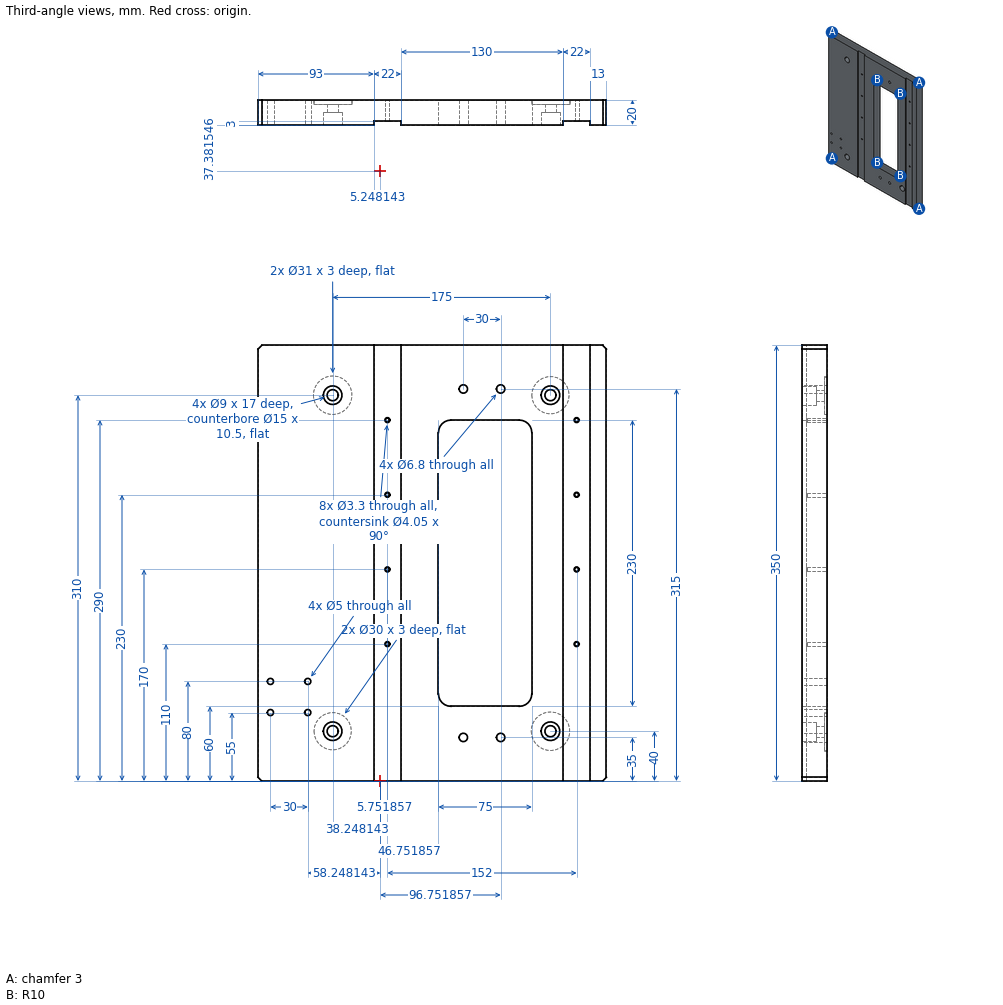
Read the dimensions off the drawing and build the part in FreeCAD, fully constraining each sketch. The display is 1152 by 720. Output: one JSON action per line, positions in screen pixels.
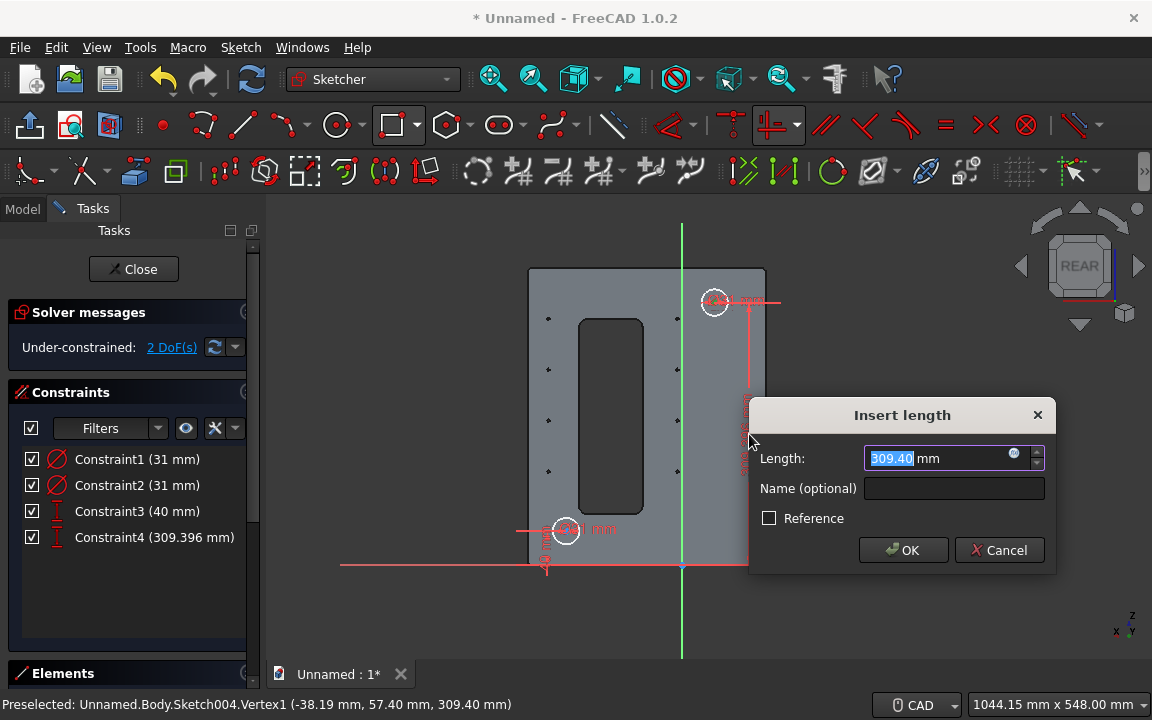
{"action": "type", "text": "310"}
{"action": "key", "text": "Return"}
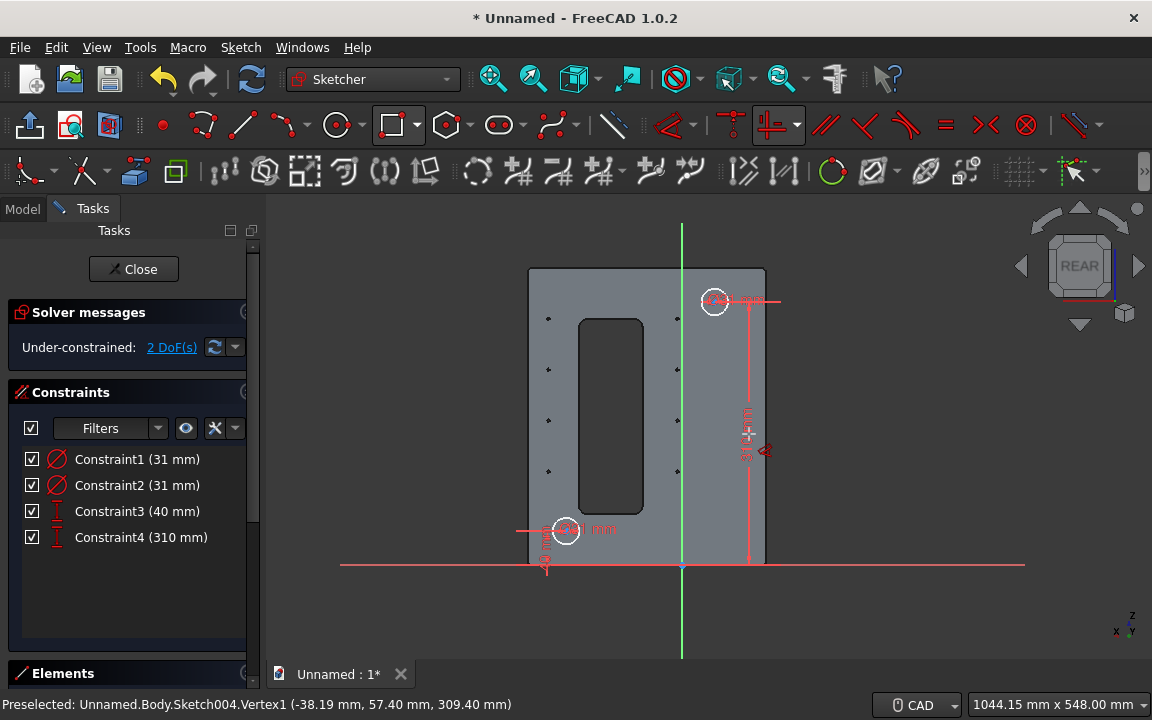
{"action": "left_click", "coordinate": [715, 302]}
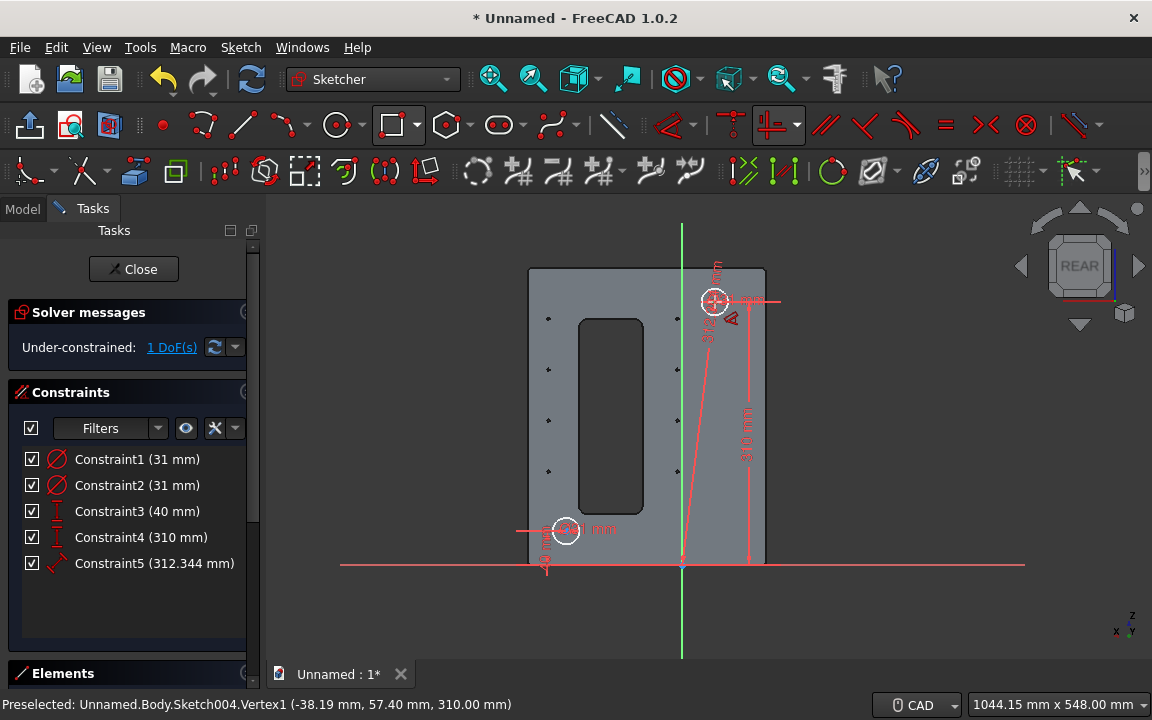
{"action": "left_click", "coordinate": [566, 531]}
{"action": "left_click", "coordinate": [640, 268]}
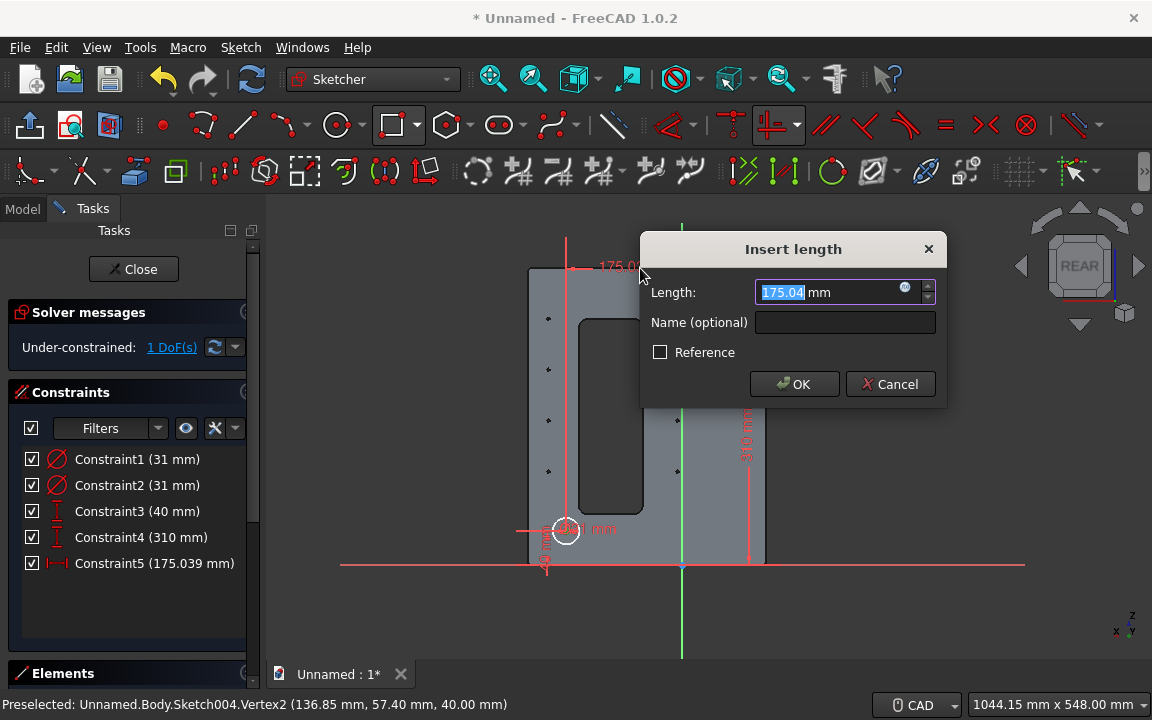
{"action": "type", "text": "175"}
{"action": "key", "text": "Return"}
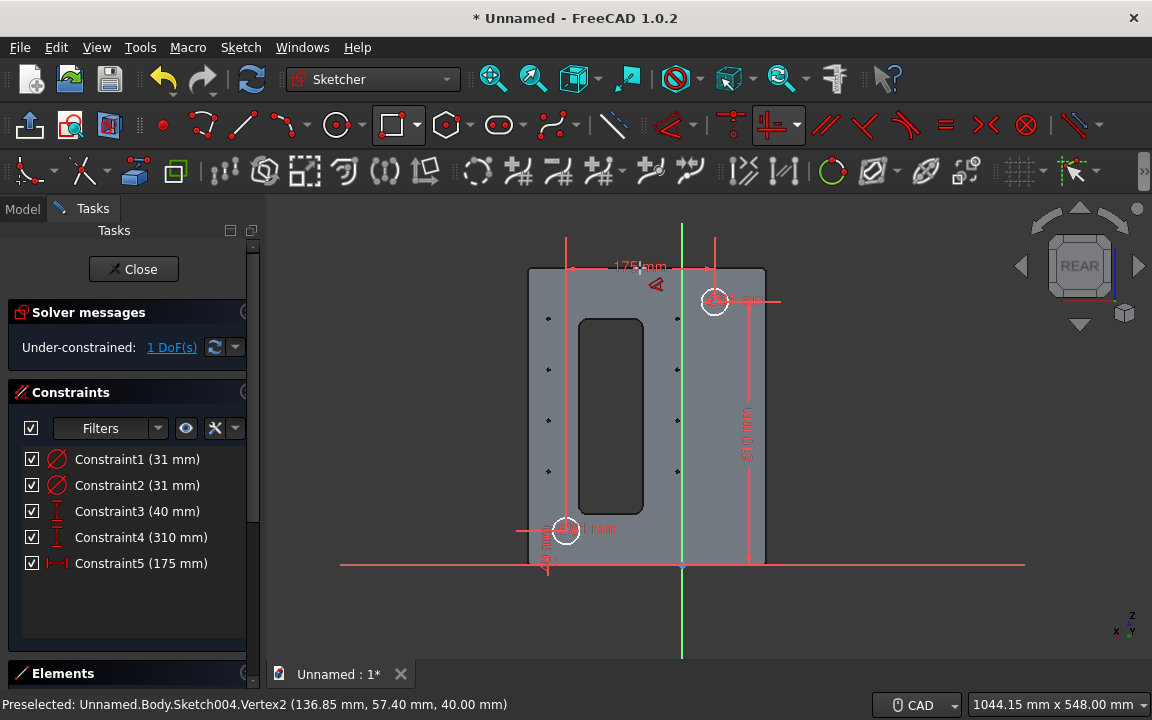
{"action": "scroll", "coordinate": [715, 302], "scroll_direction": "up", "scroll_amount": 2}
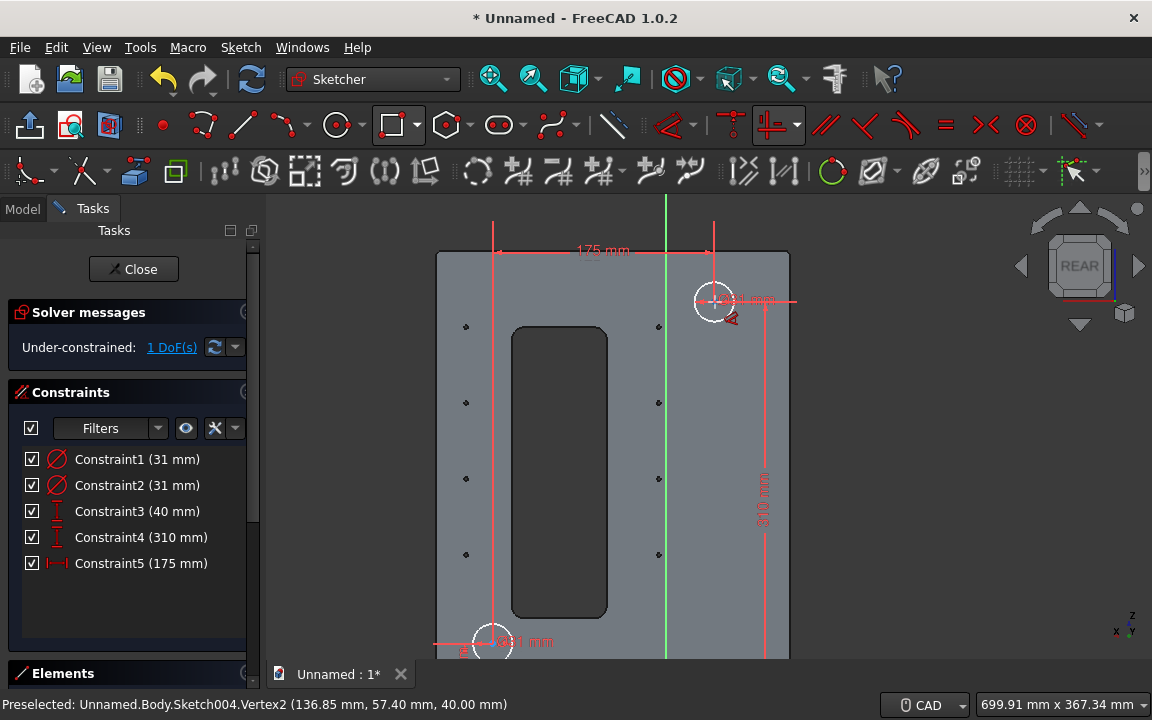
{"action": "left_click", "coordinate": [714, 302]}
{"action": "left_click", "coordinate": [690, 268]}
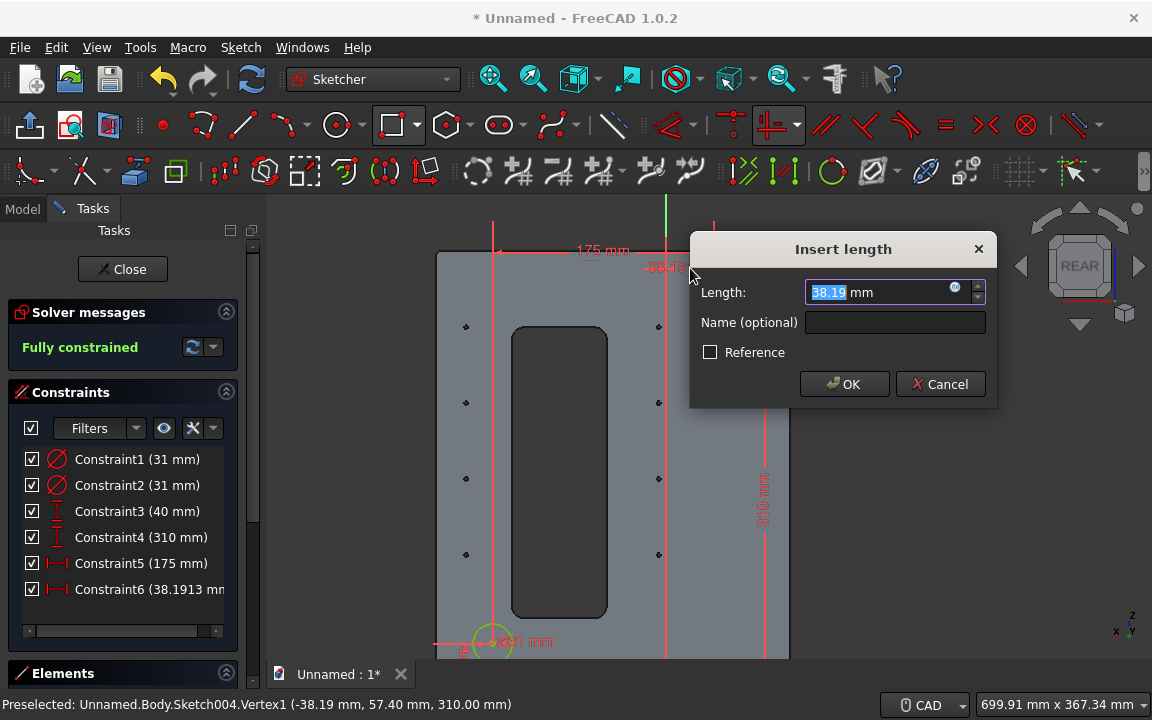
{"action": "type", "text": "38.248143"}
{"action": "key", "text": "Return"}
{"action": "key", "text": "Escape"}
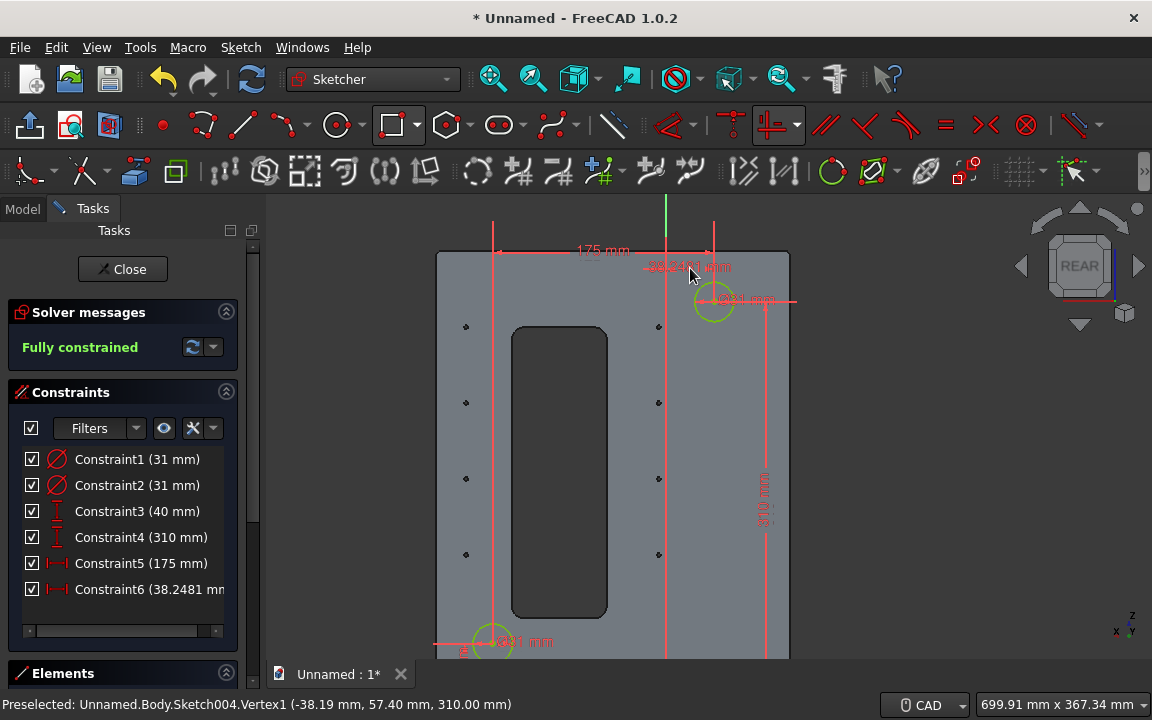
{"action": "left_click", "coordinate": [123, 269]}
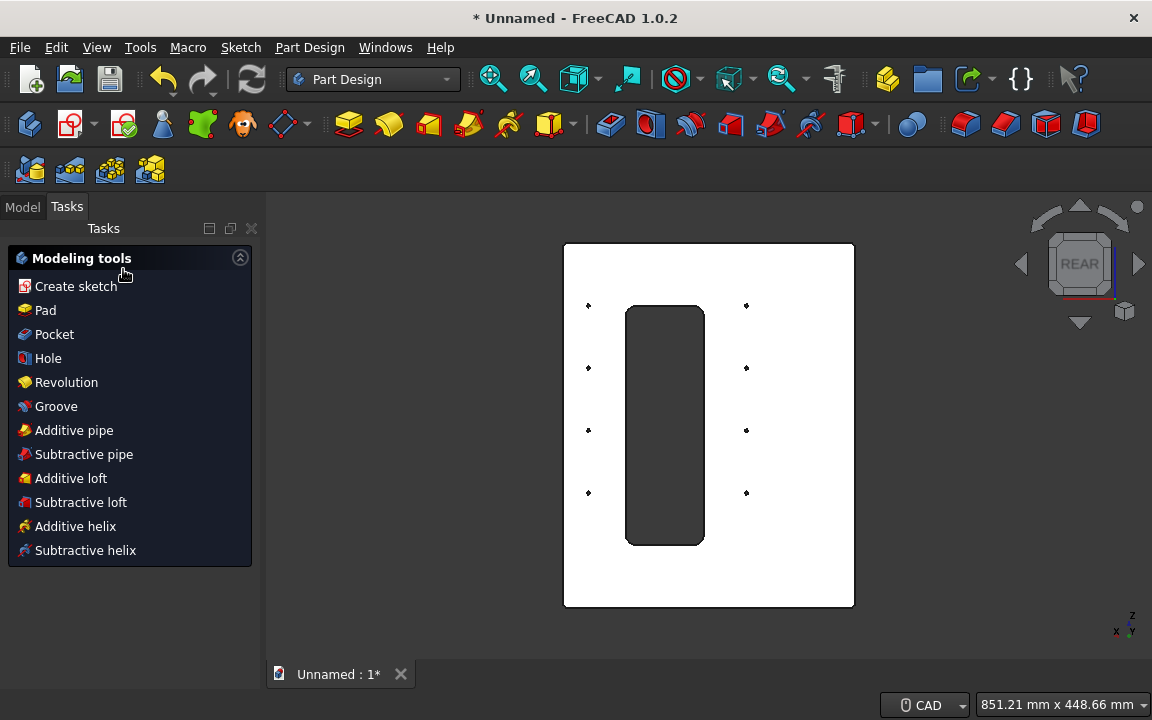
{"action": "left_click", "coordinate": [652, 124]}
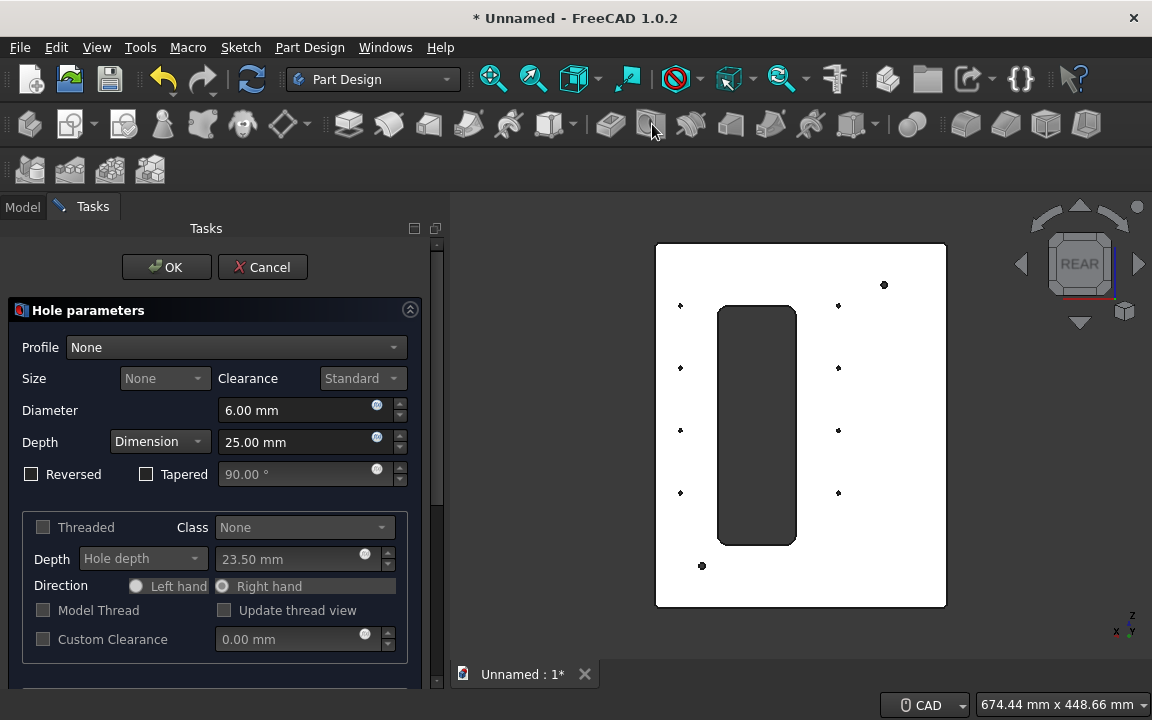
{"action": "triple_click", "coordinate": [305, 410]}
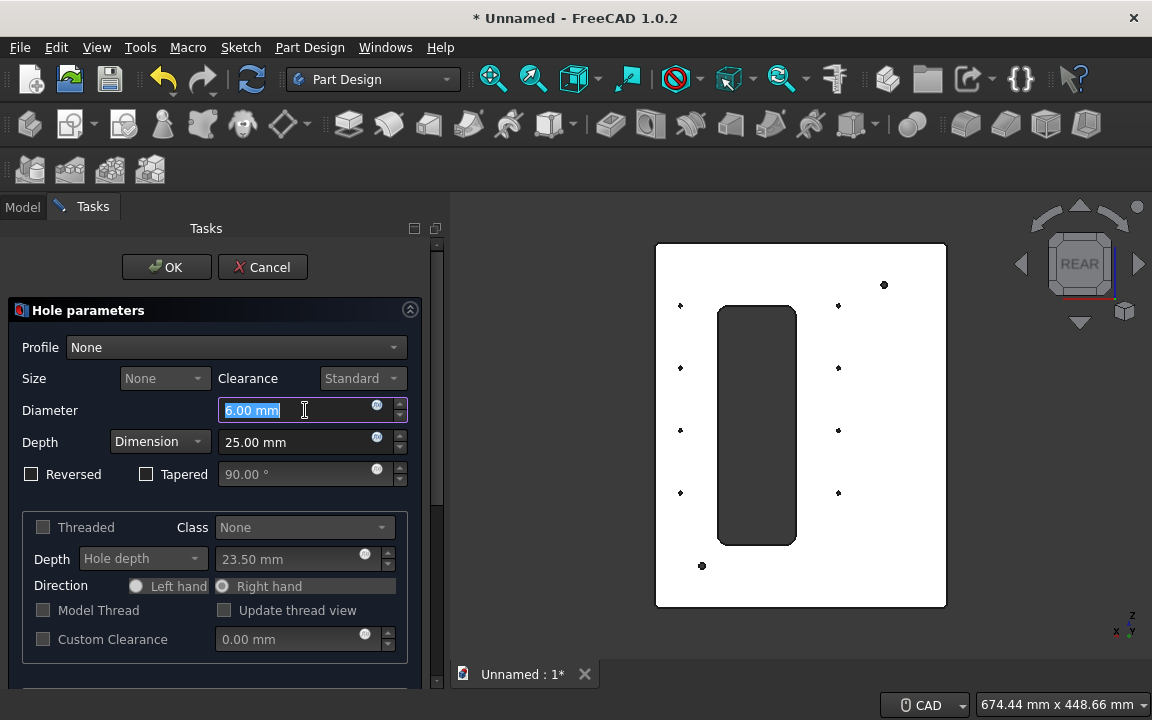
{"action": "type", "text": "31"}
{"action": "key", "text": "Tab"}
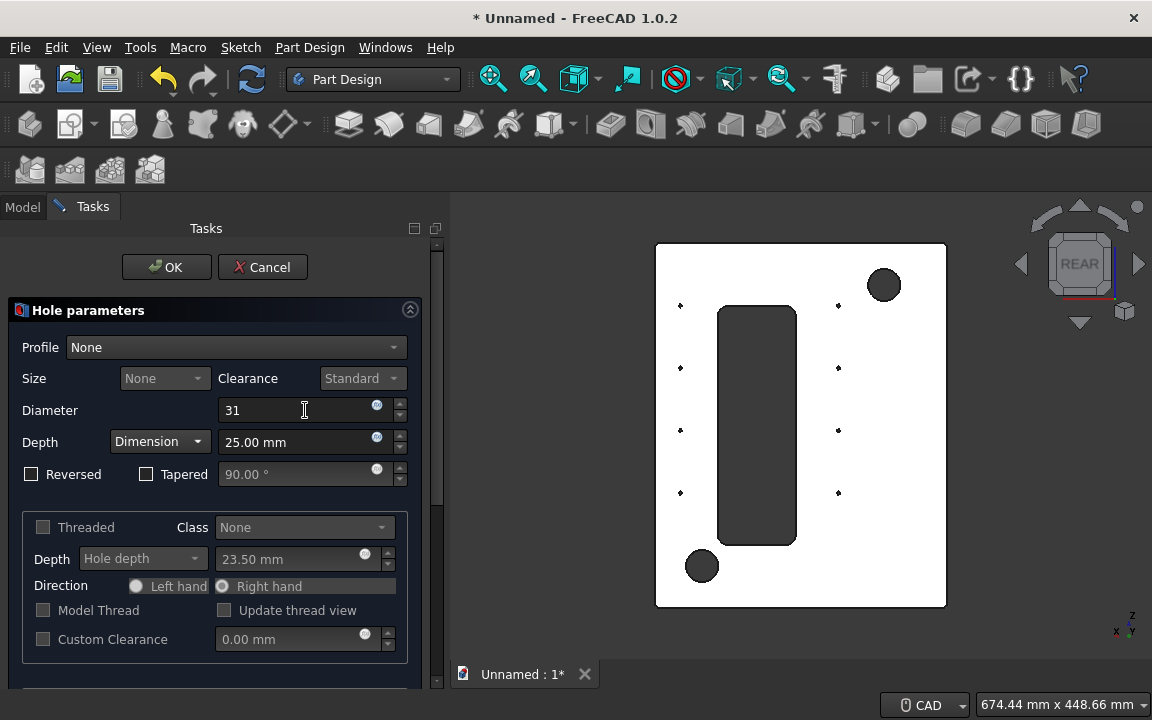
{"action": "triple_click", "coordinate": [305, 442]}